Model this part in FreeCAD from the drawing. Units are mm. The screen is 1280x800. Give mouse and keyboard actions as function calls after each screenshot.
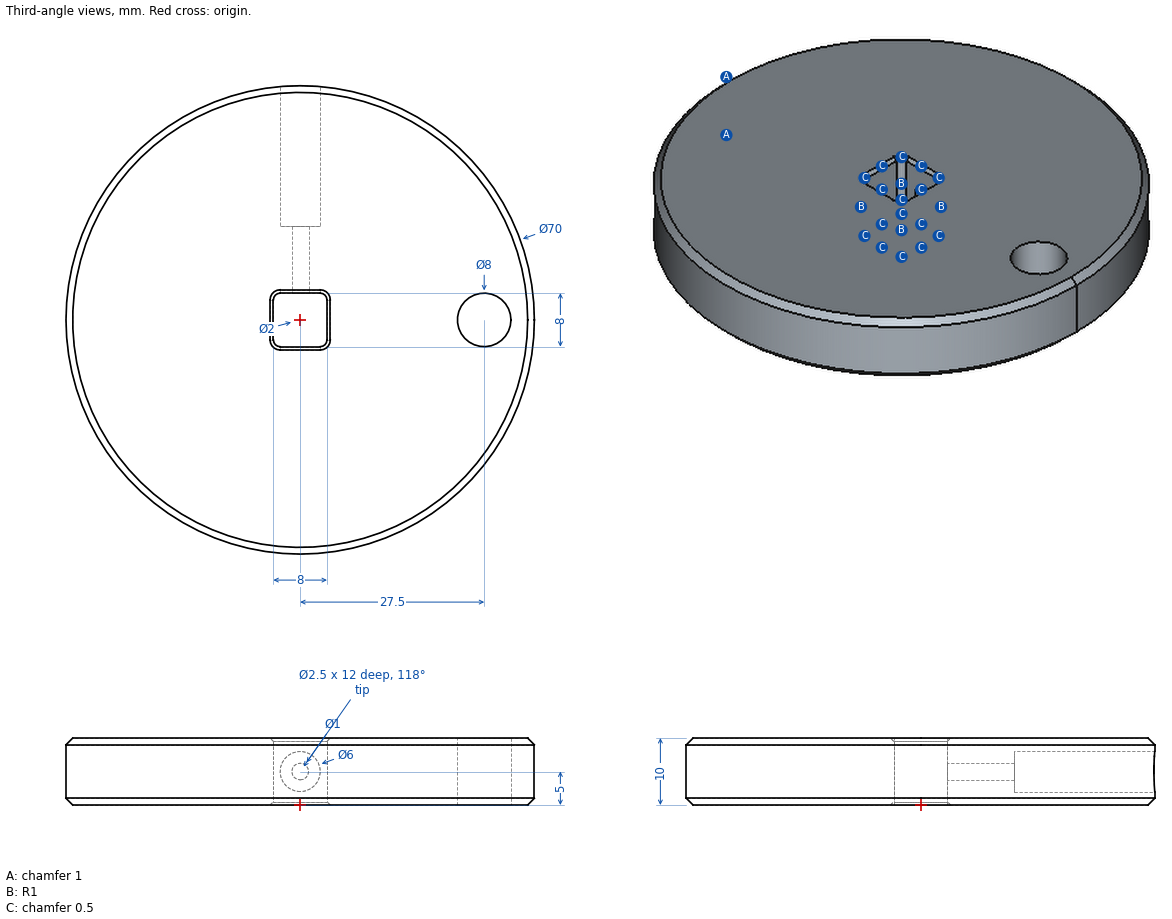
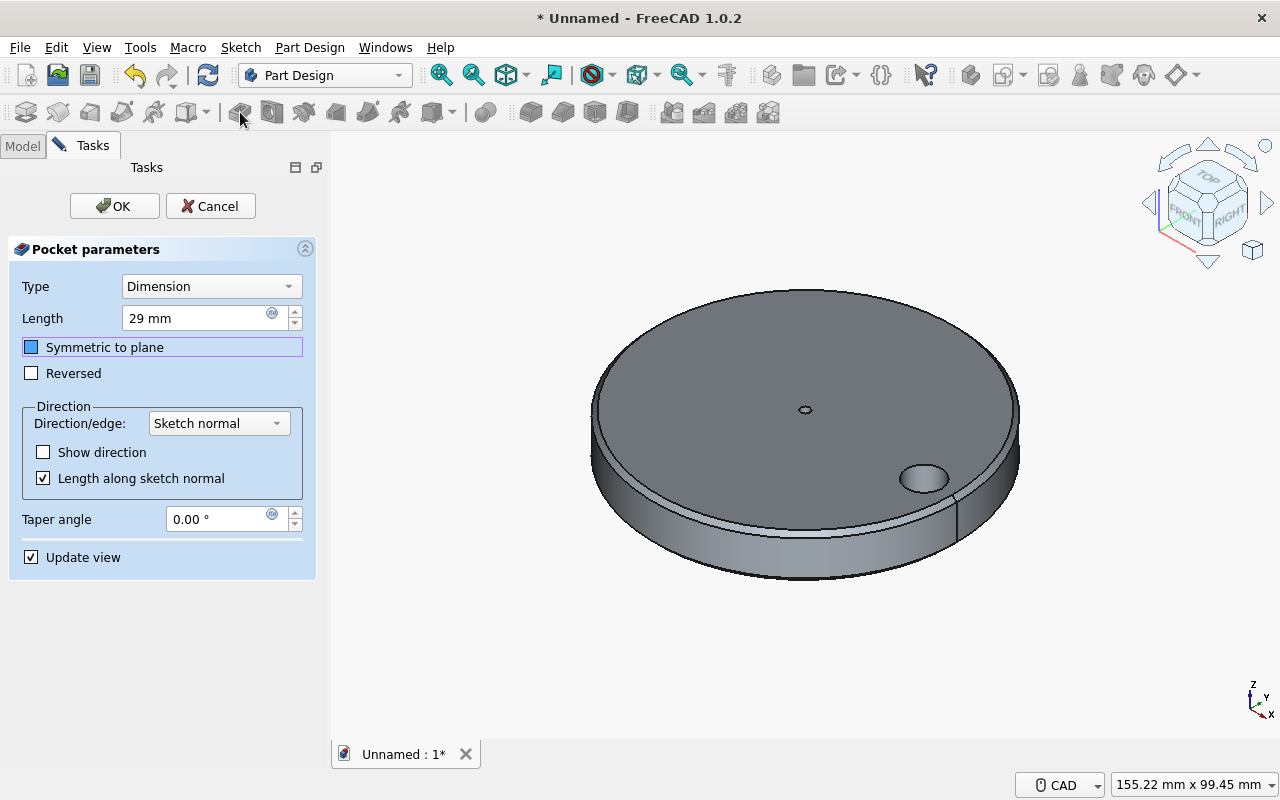
click(115, 206)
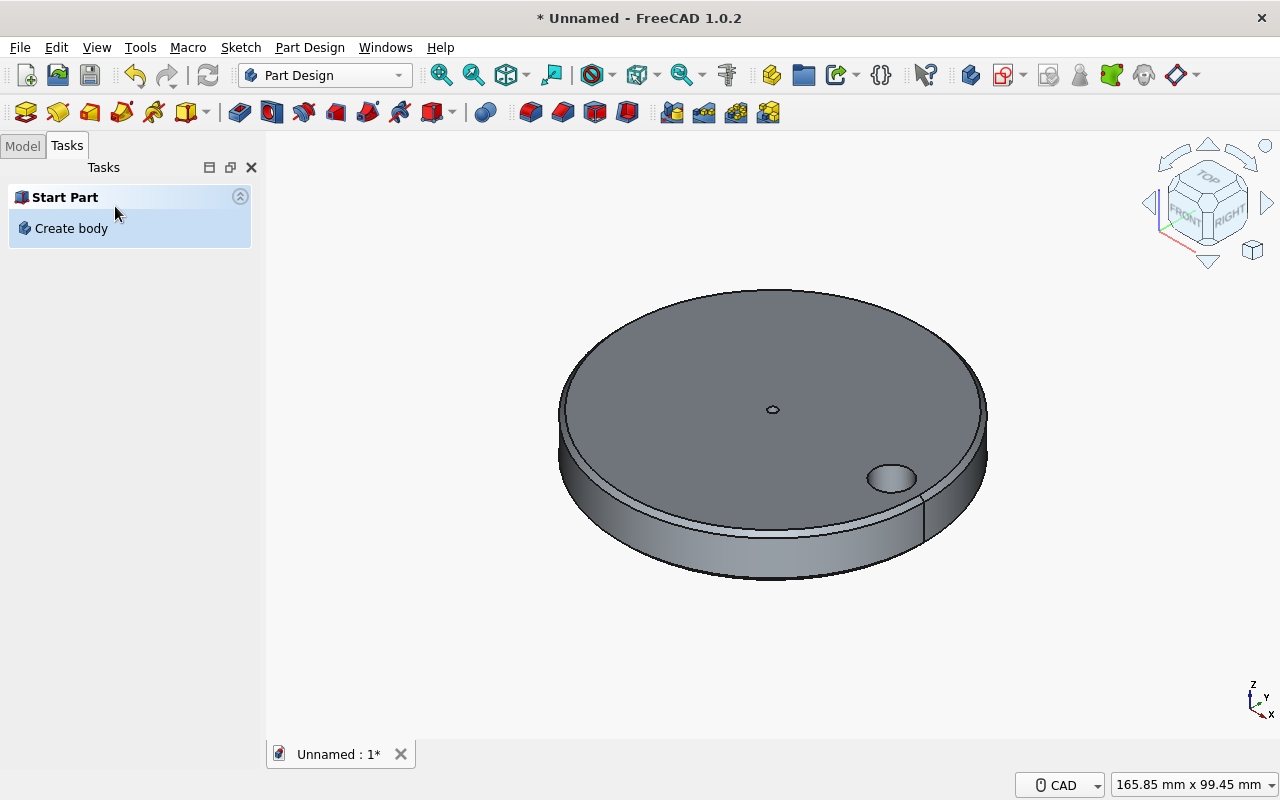
click(689, 457)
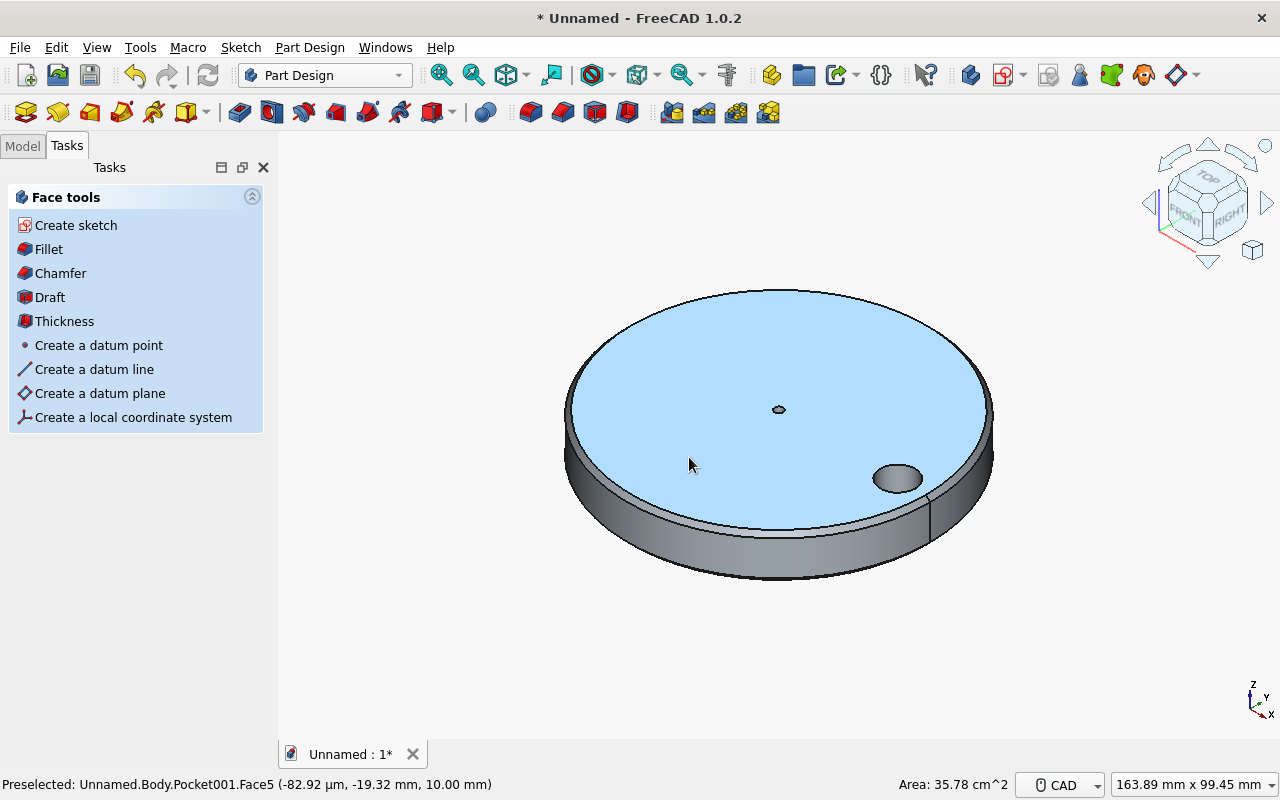
click(1004, 76)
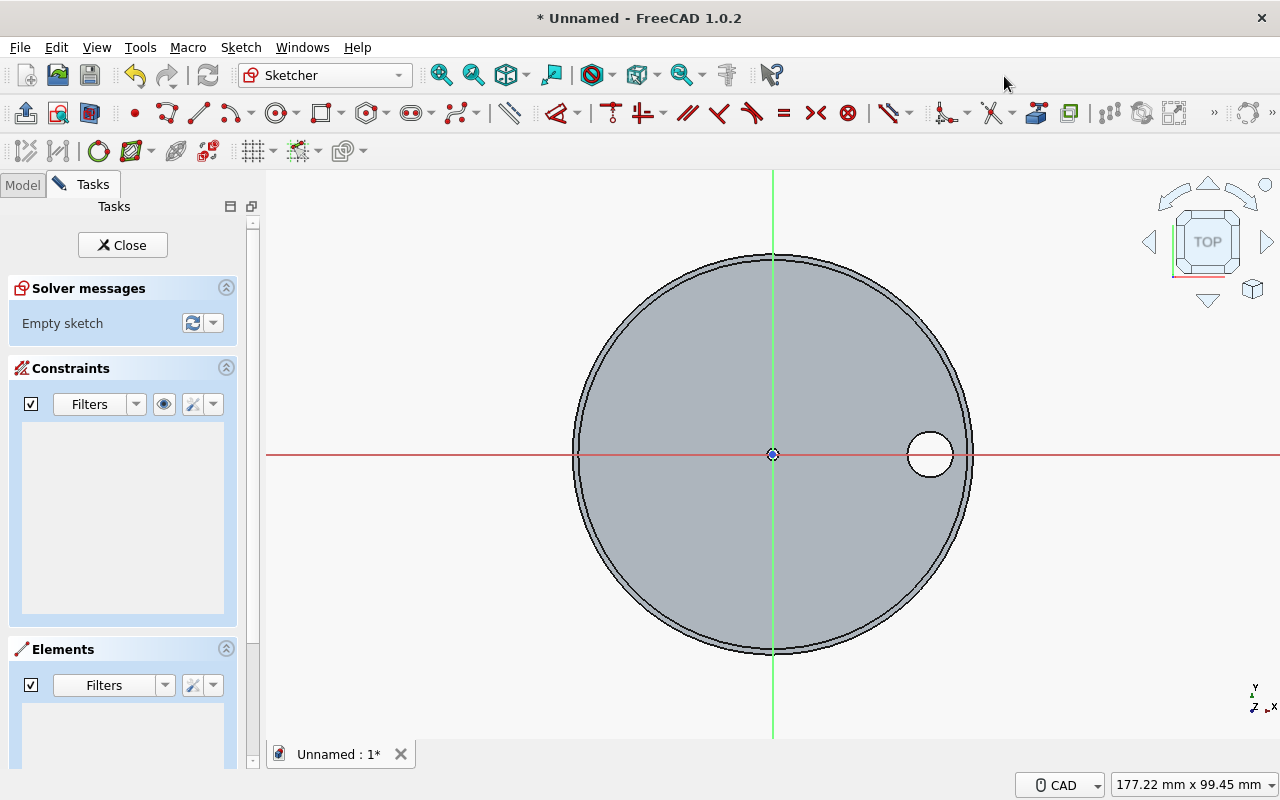
scroll(784, 454, up, 10)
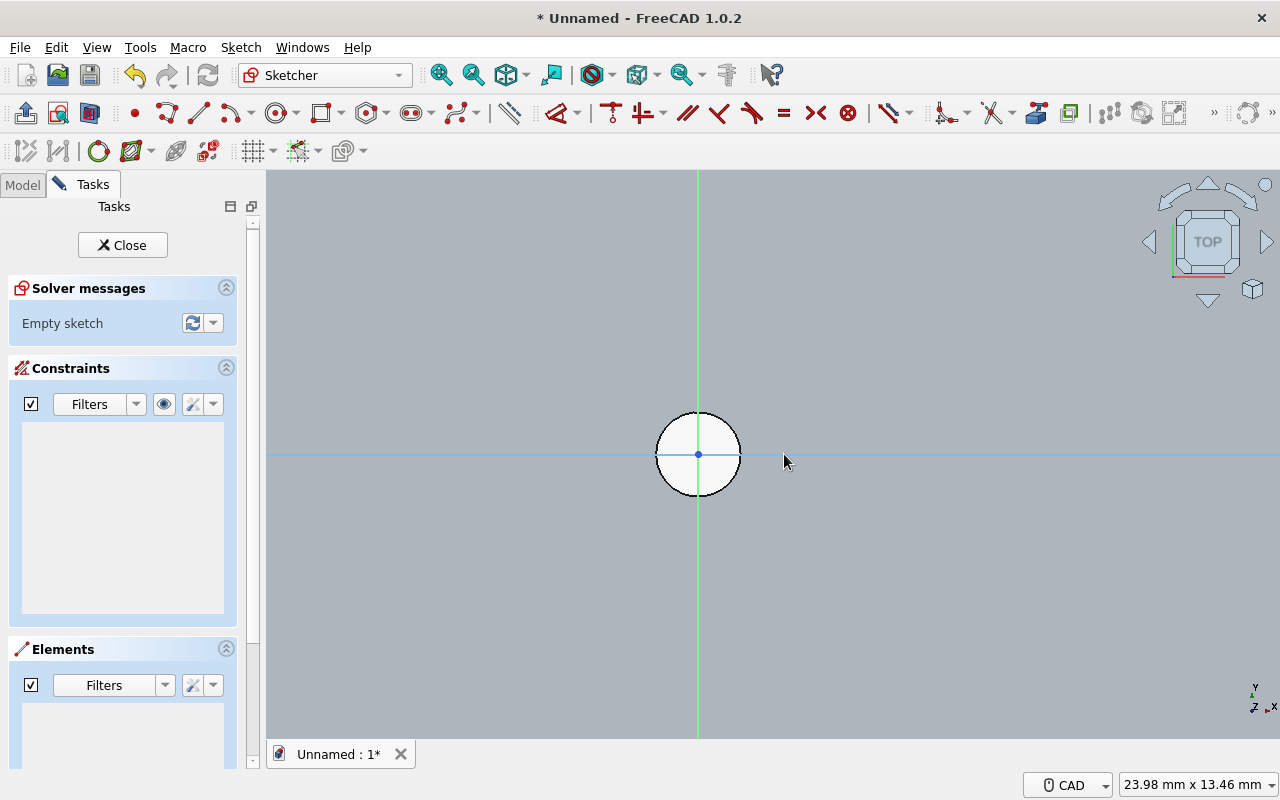
click(344, 114)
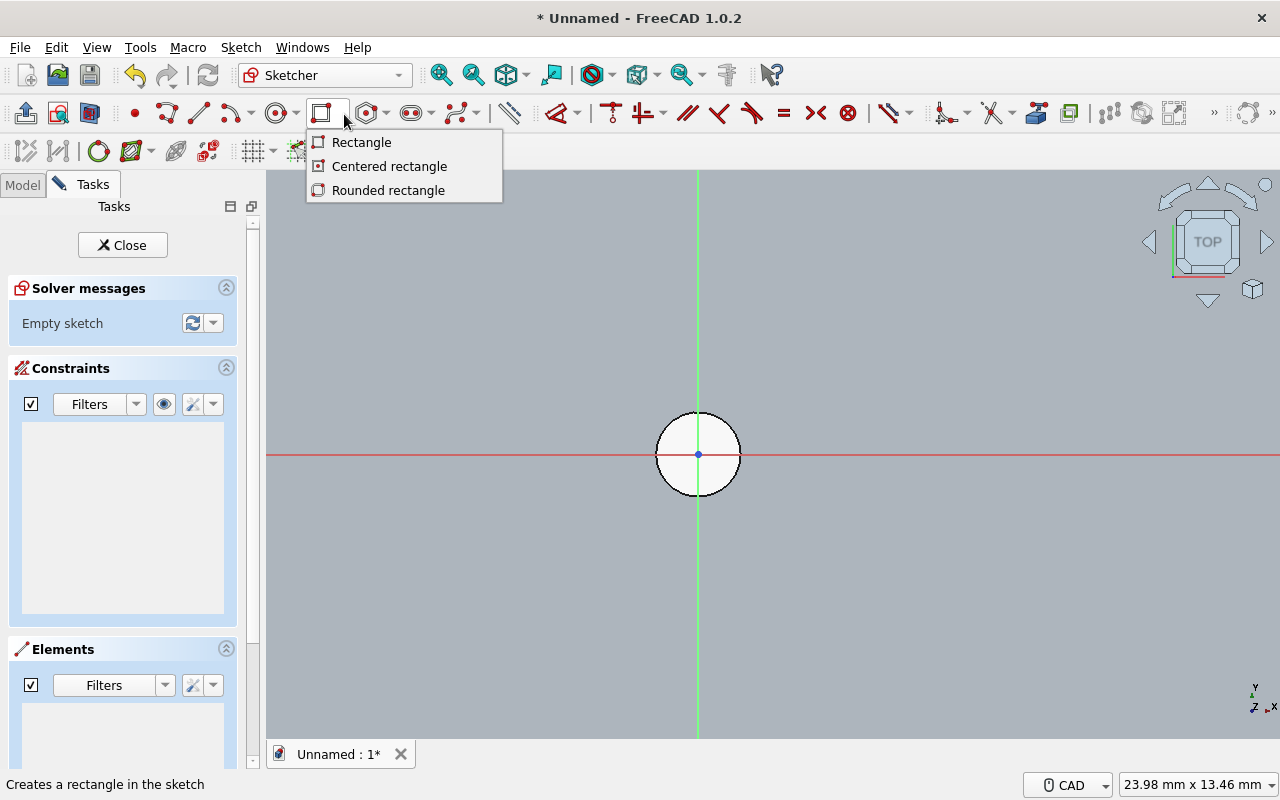
click(404, 166)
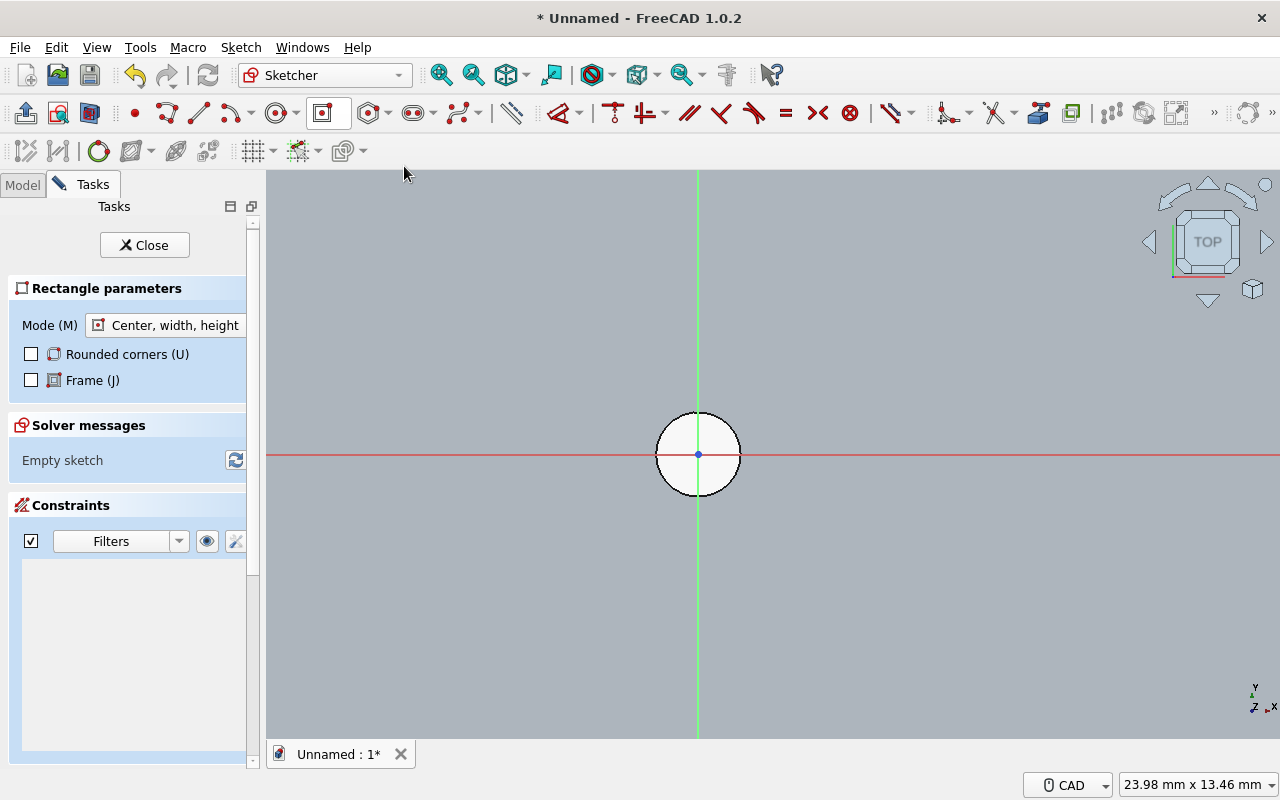
click(698, 454)
click(868, 285)
key(Escape)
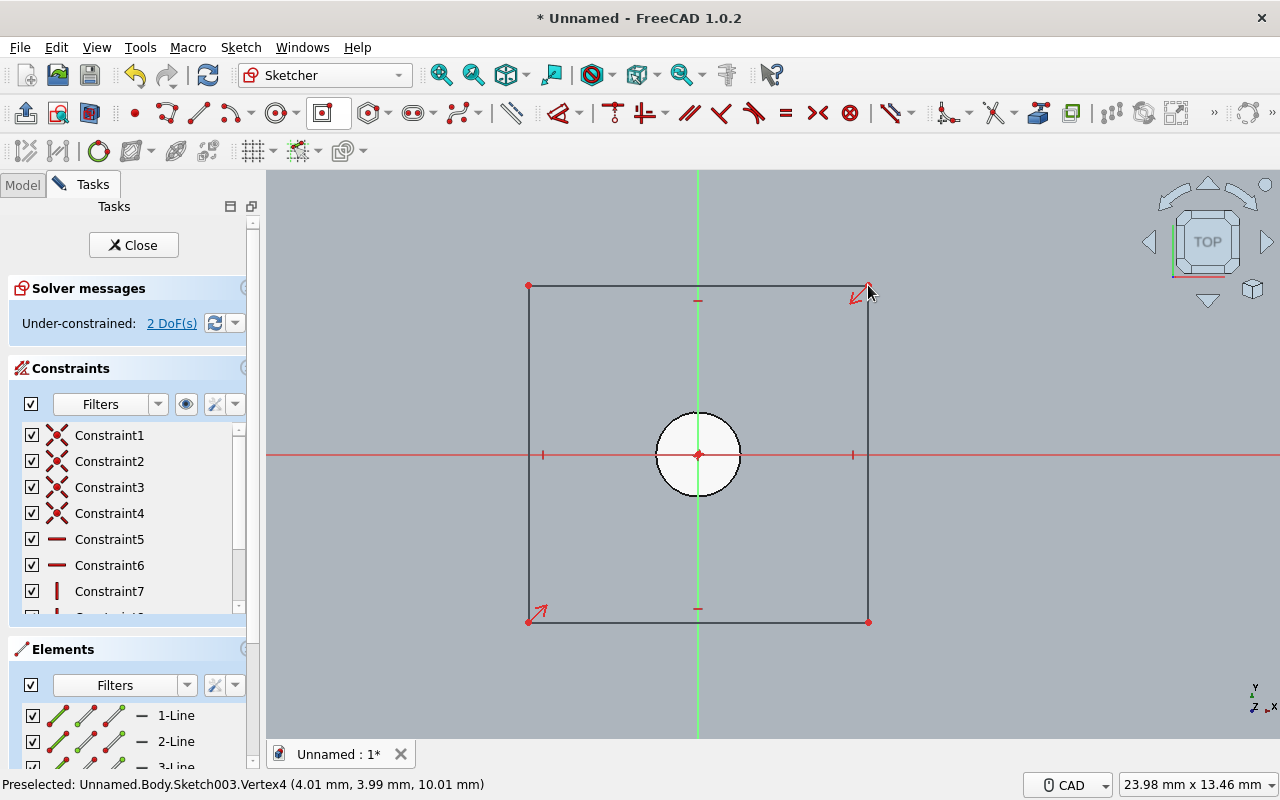
key(d)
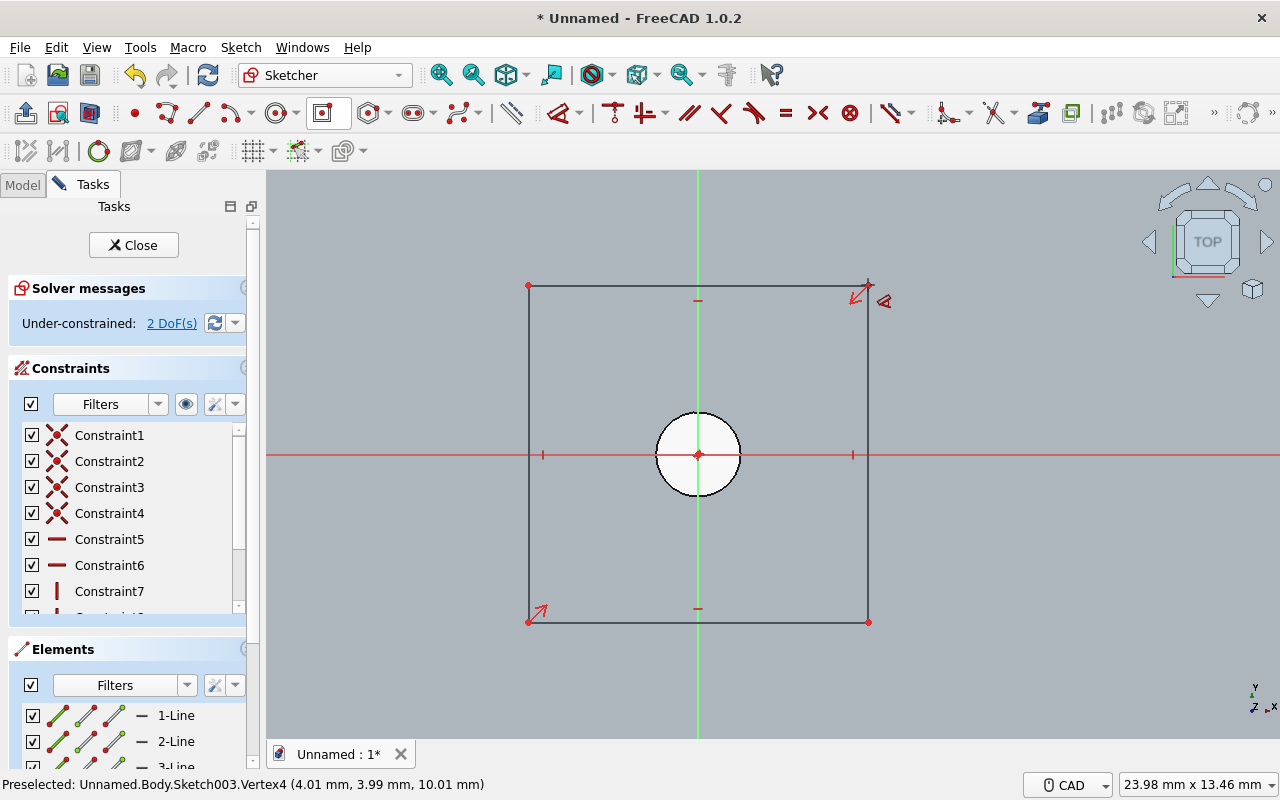
click(631, 623)
click(620, 657)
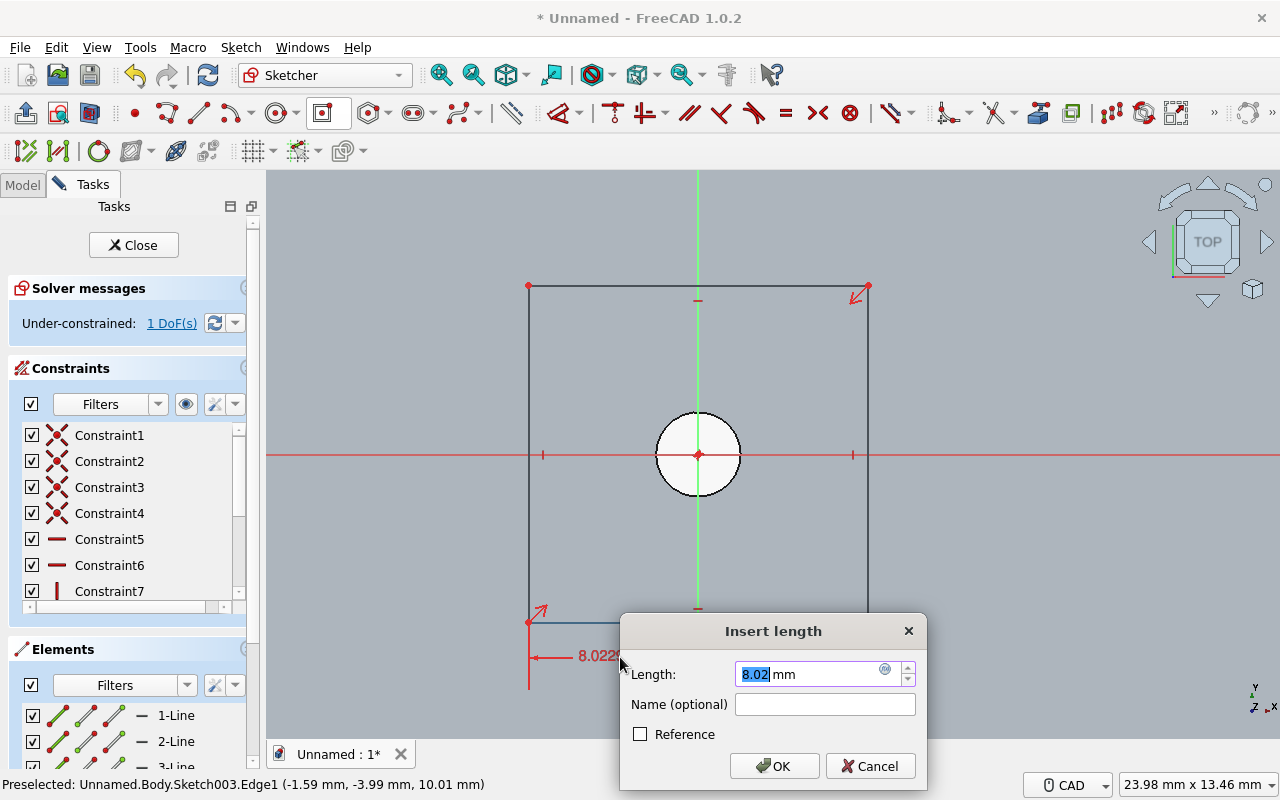
text(8)
key(Return)